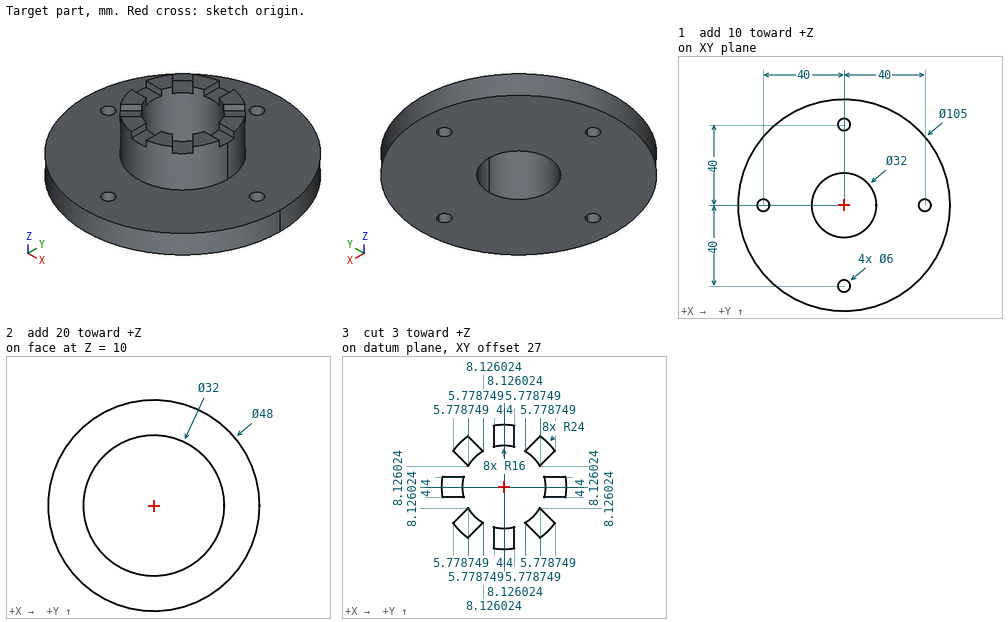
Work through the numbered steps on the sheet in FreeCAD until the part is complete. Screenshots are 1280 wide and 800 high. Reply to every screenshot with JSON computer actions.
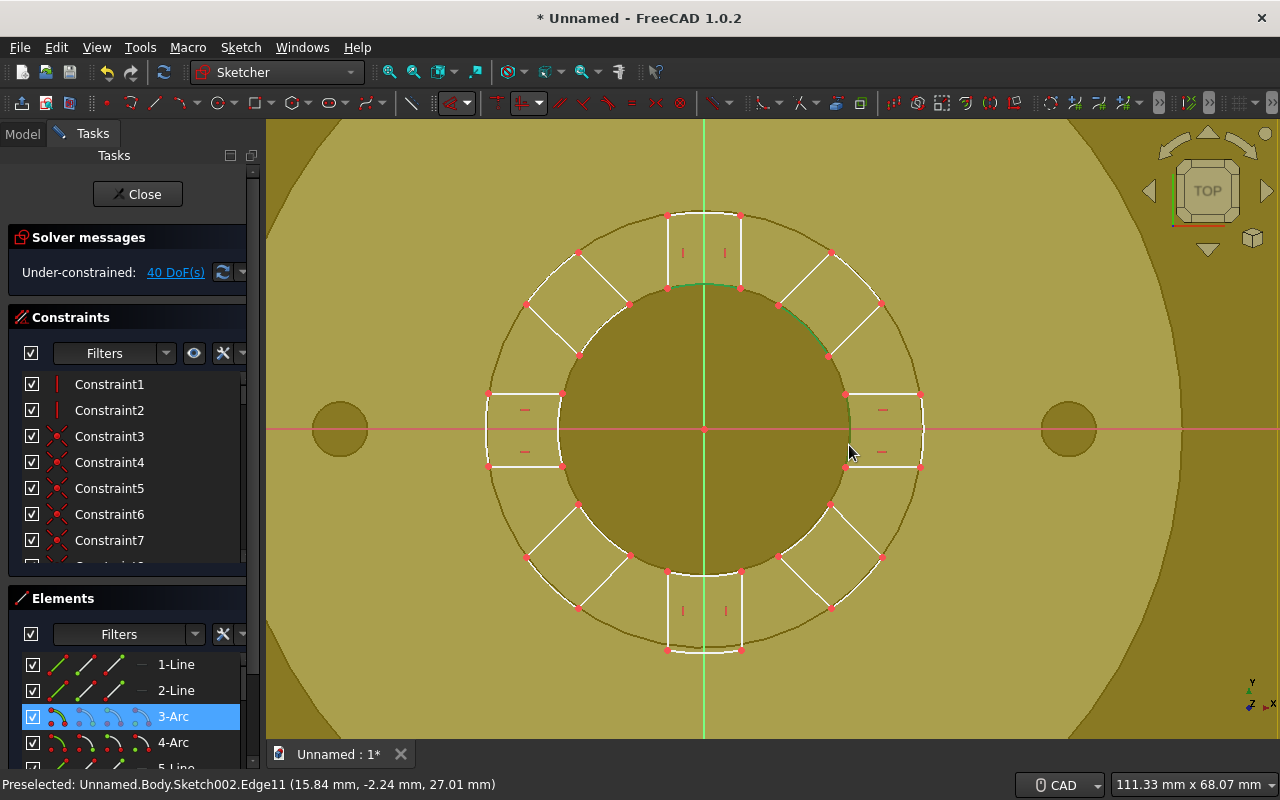
{"action": "left_click", "coordinate": [797, 544]}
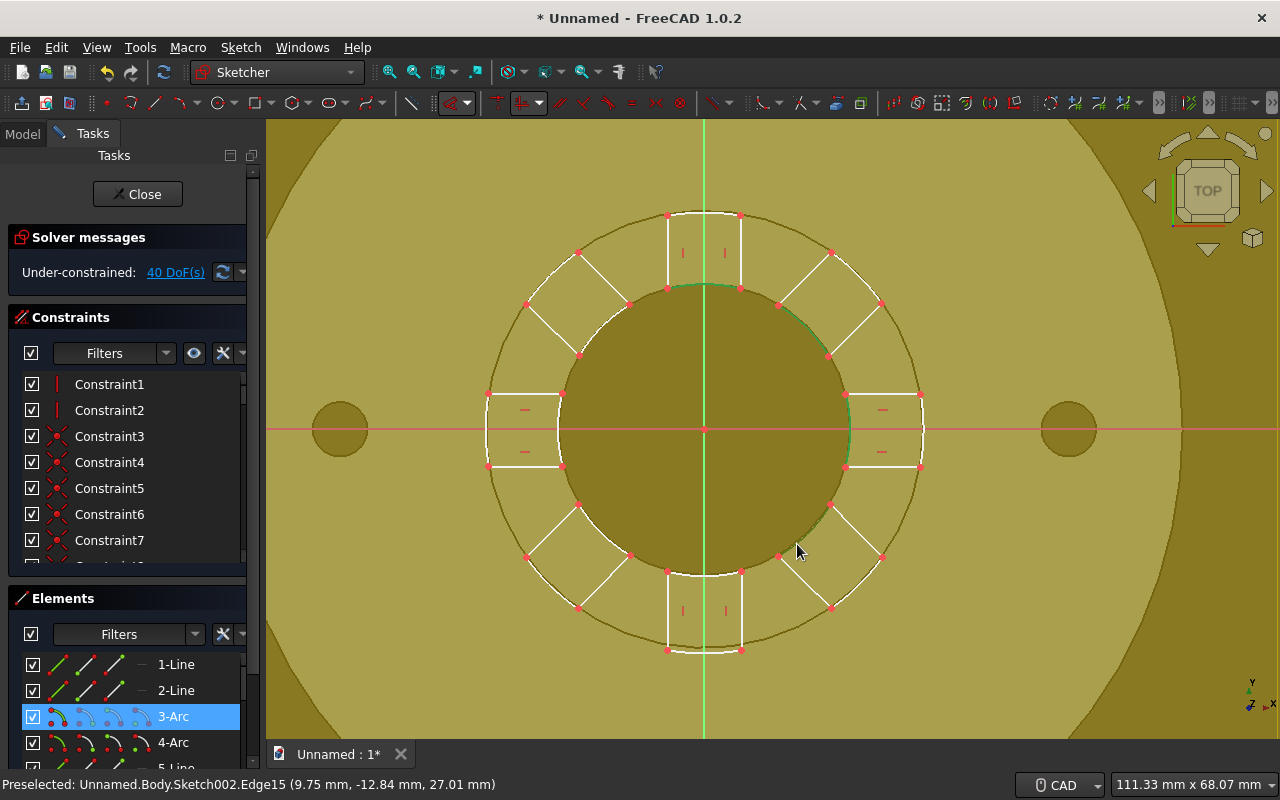
{"action": "left_click", "coordinate": [690, 576]}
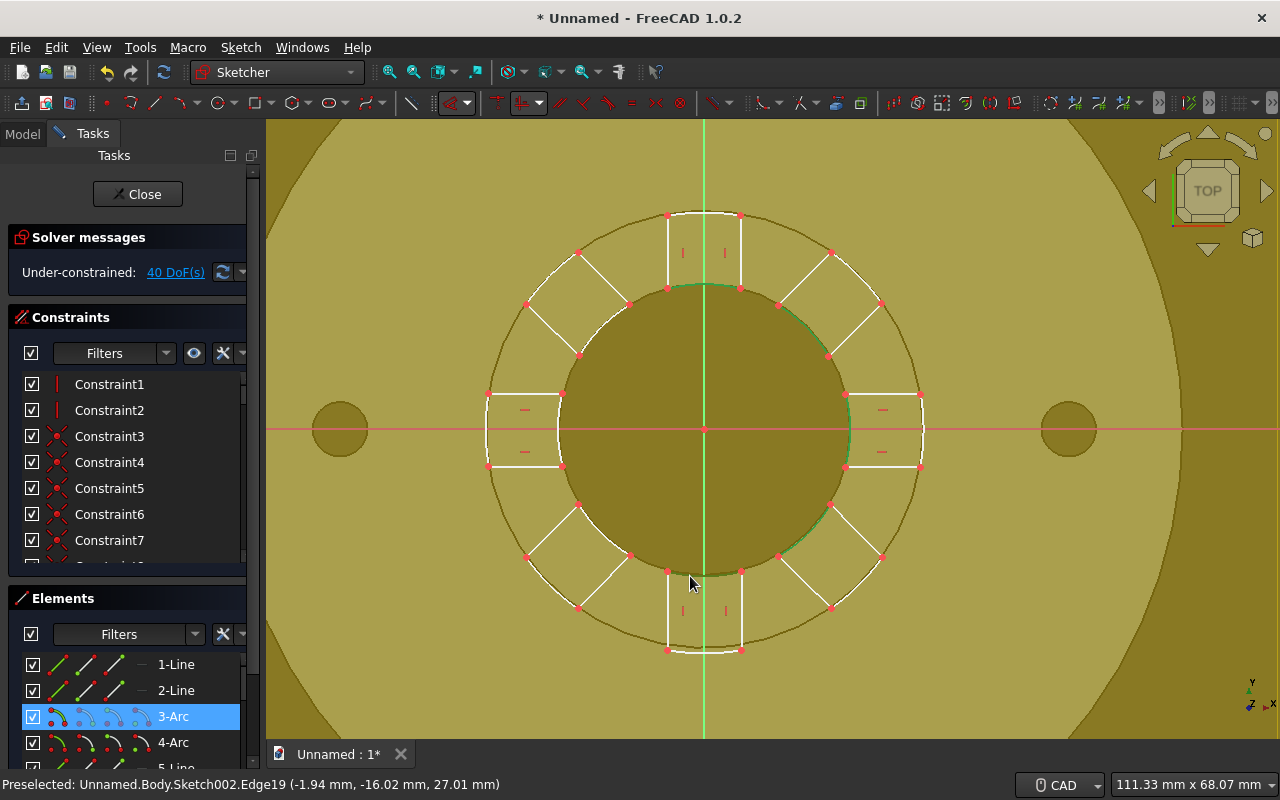
{"action": "left_click", "coordinate": [591, 522]}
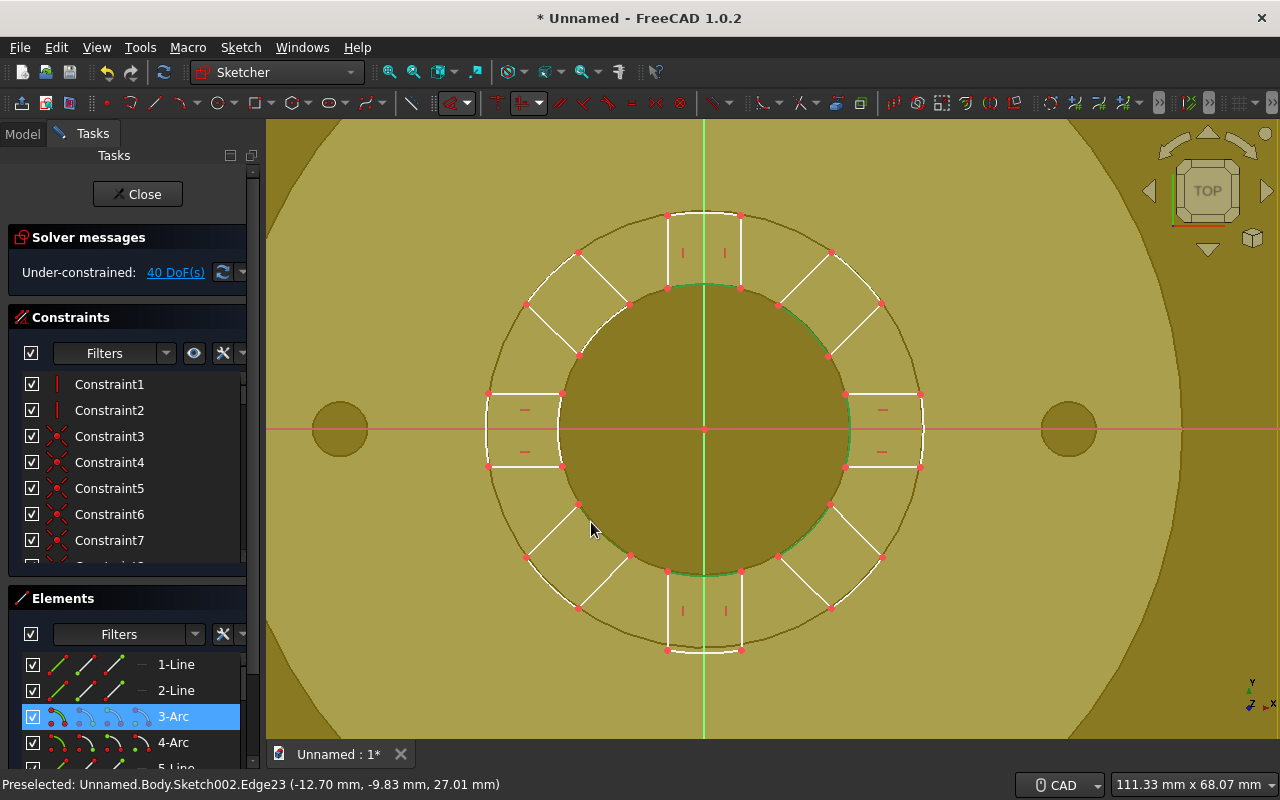
{"action": "left_click", "coordinate": [559, 416]}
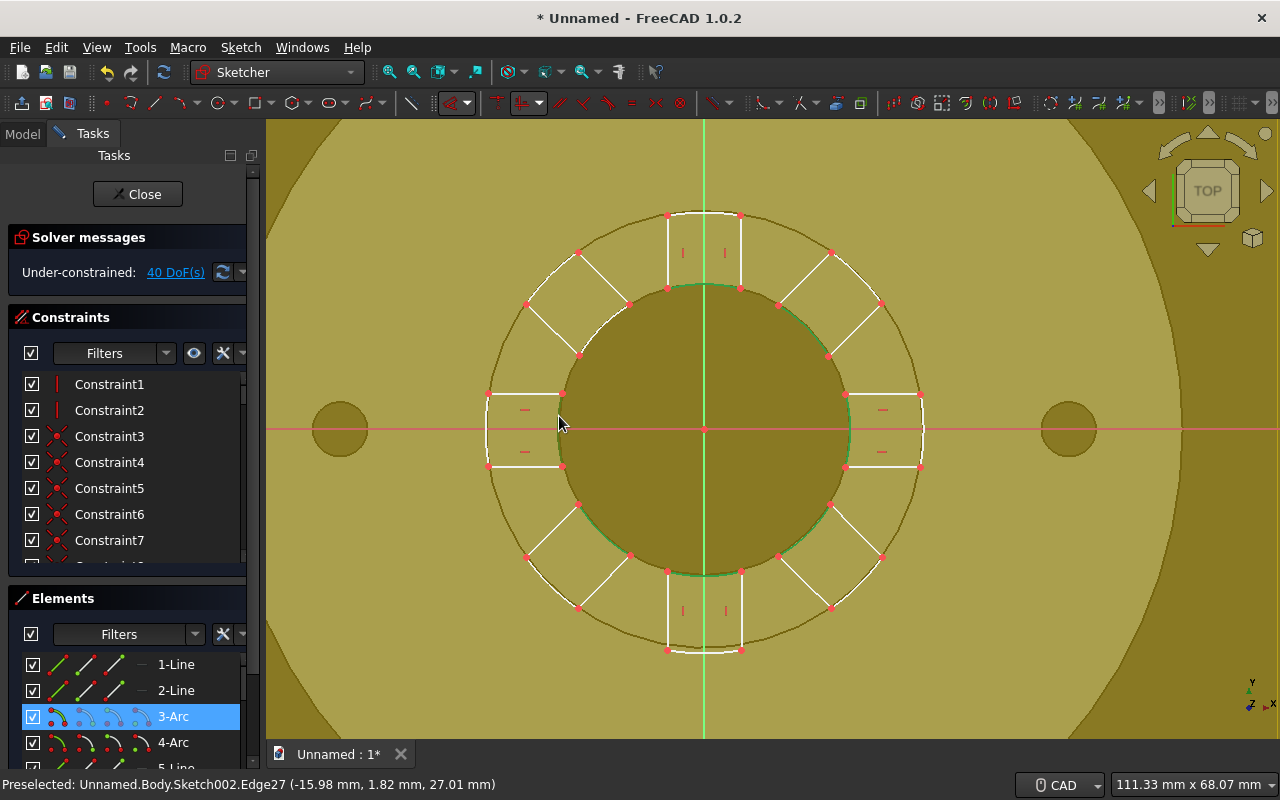
{"action": "left_click", "coordinate": [612, 317]}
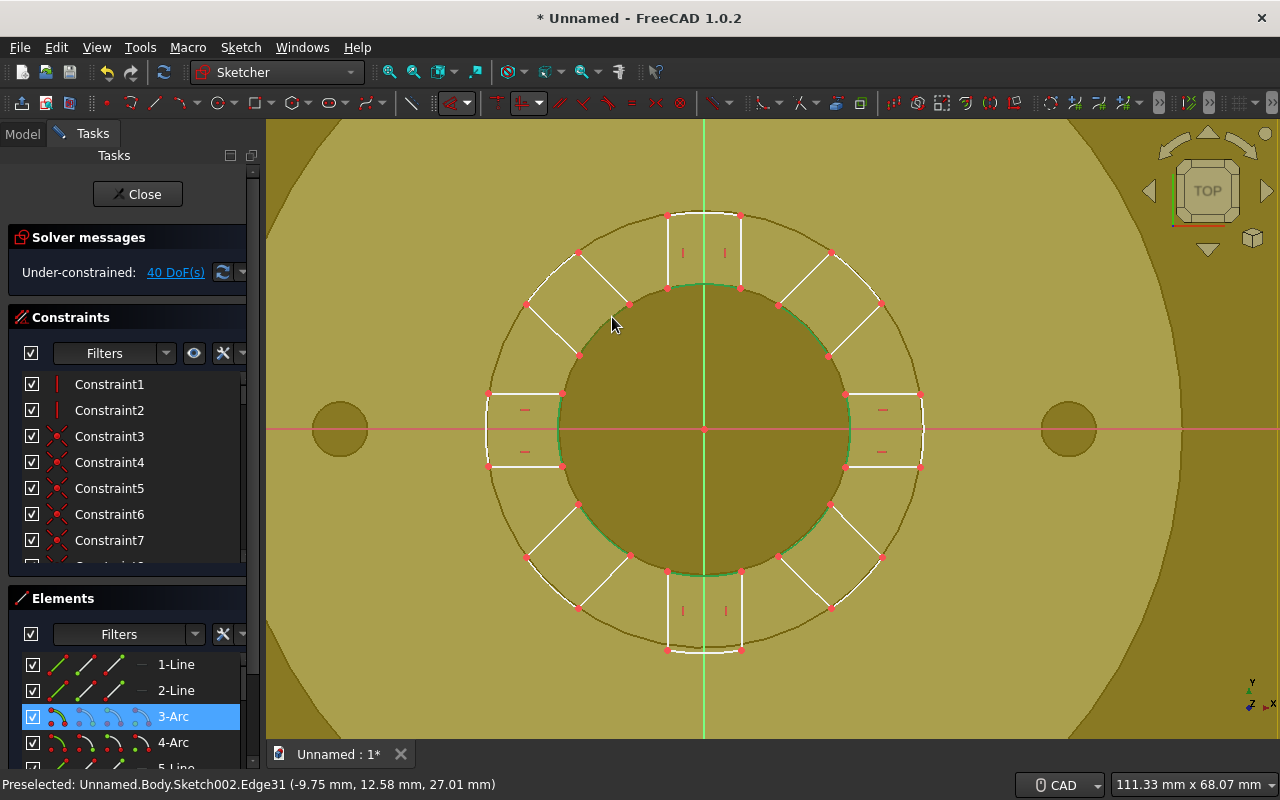
{"action": "left_click", "coordinate": [632, 104]}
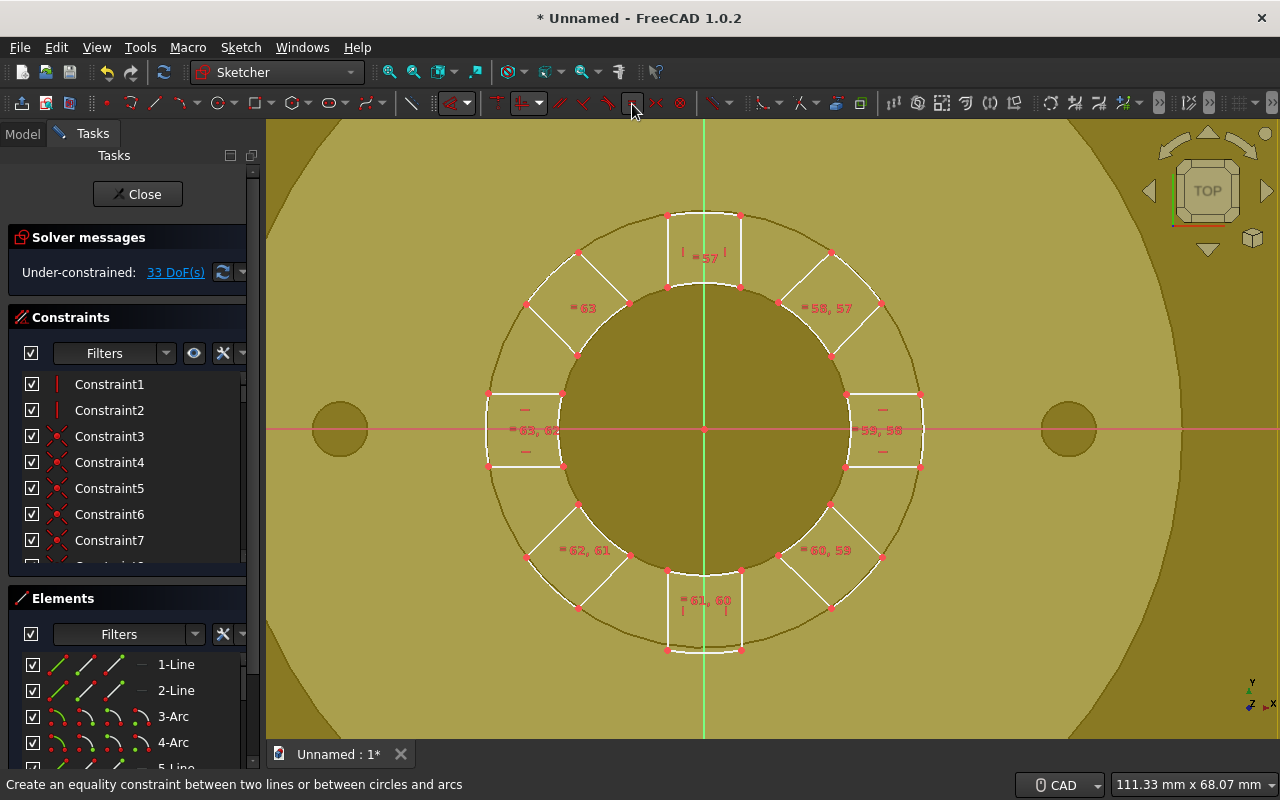
{"action": "left_click", "coordinate": [719, 213]}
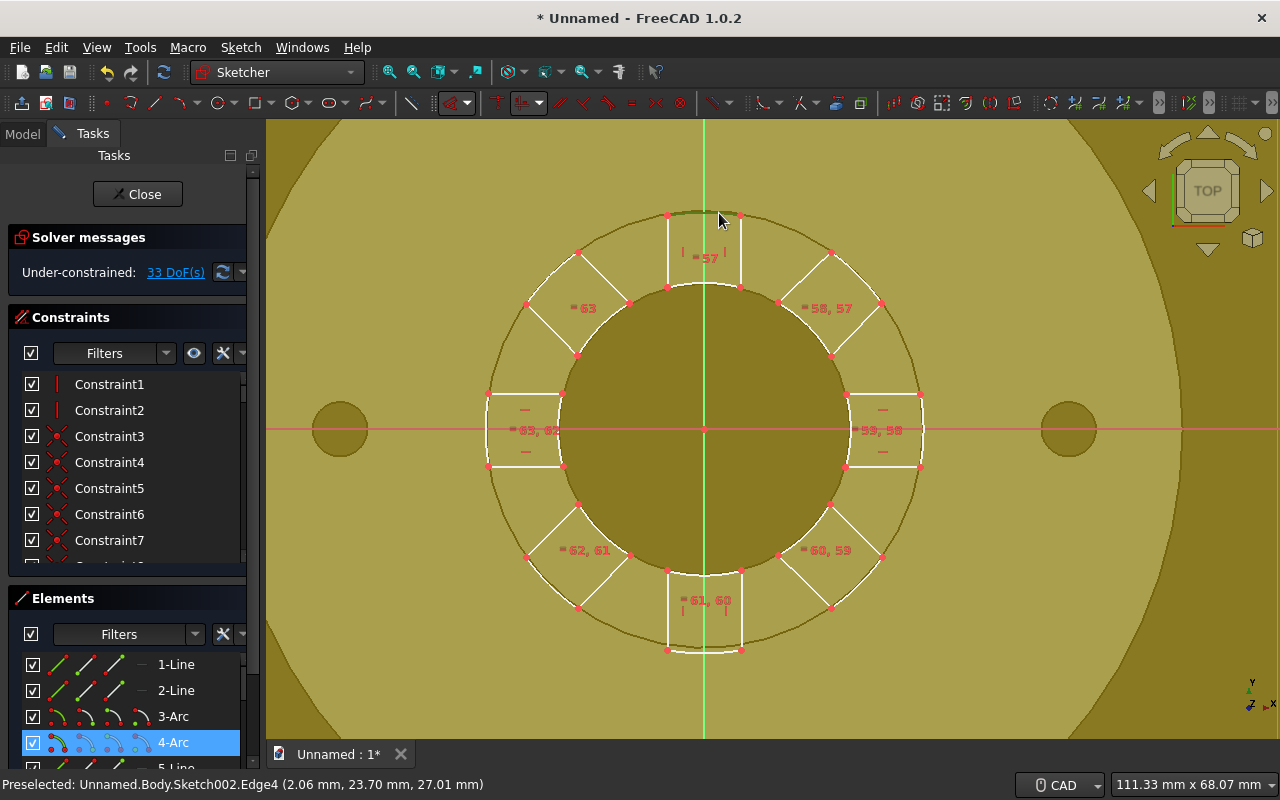
{"action": "left_click", "coordinate": [868, 286]}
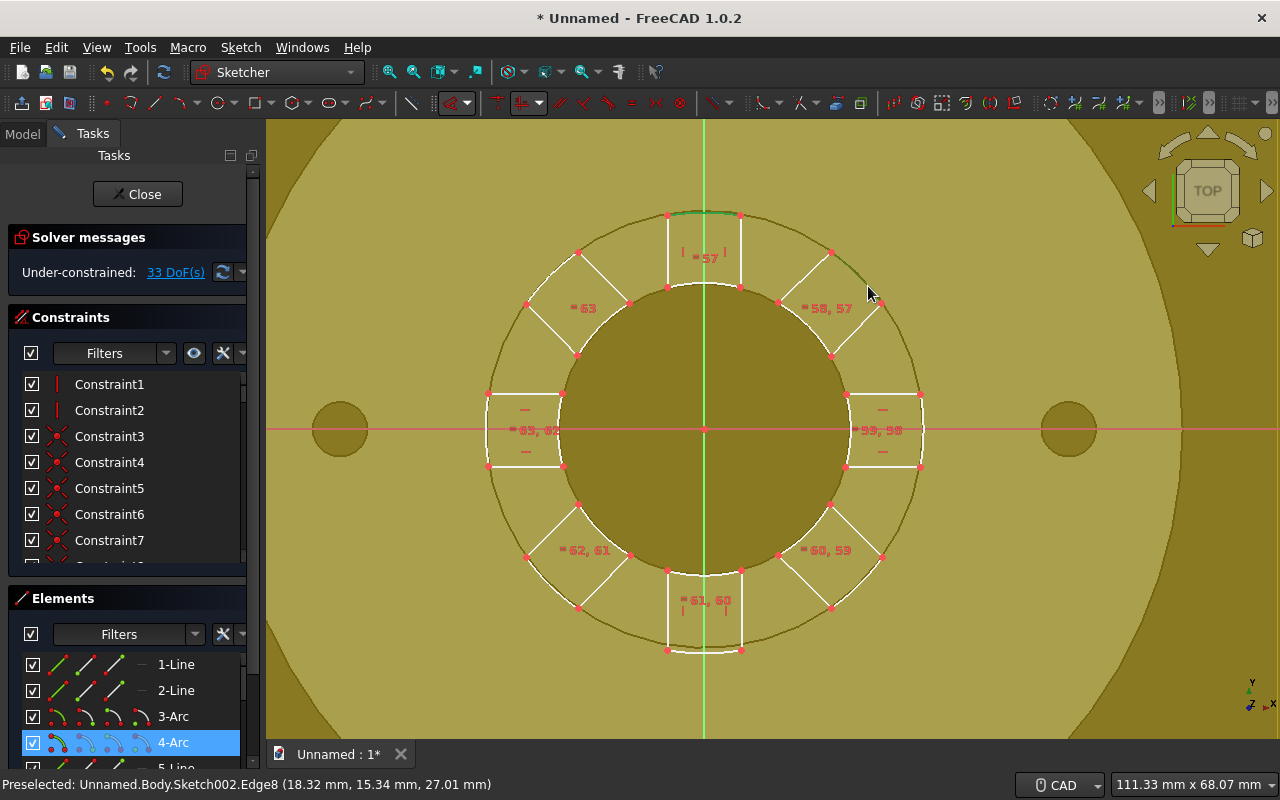
{"action": "left_click", "coordinate": [923, 445]}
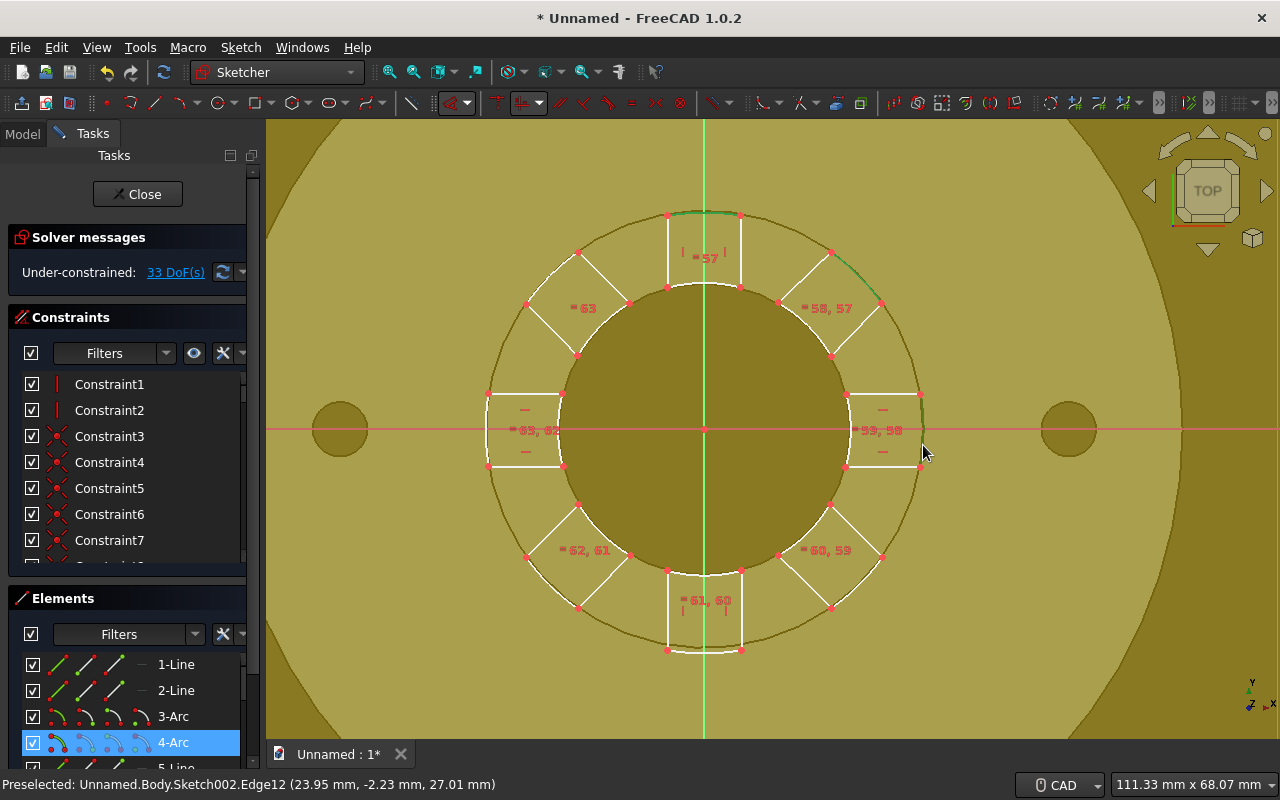
{"action": "left_click", "coordinate": [848, 595]}